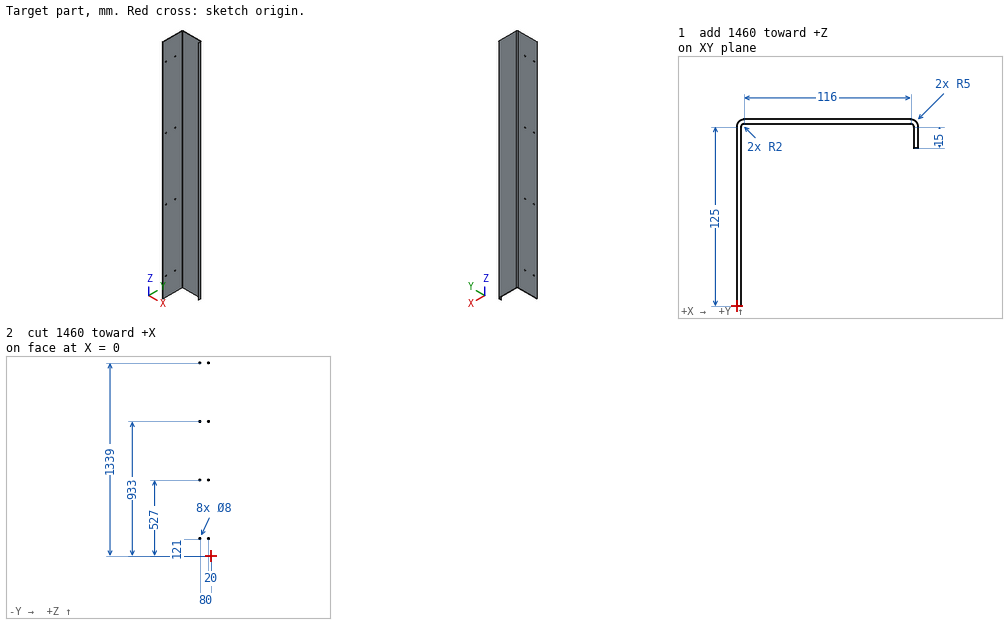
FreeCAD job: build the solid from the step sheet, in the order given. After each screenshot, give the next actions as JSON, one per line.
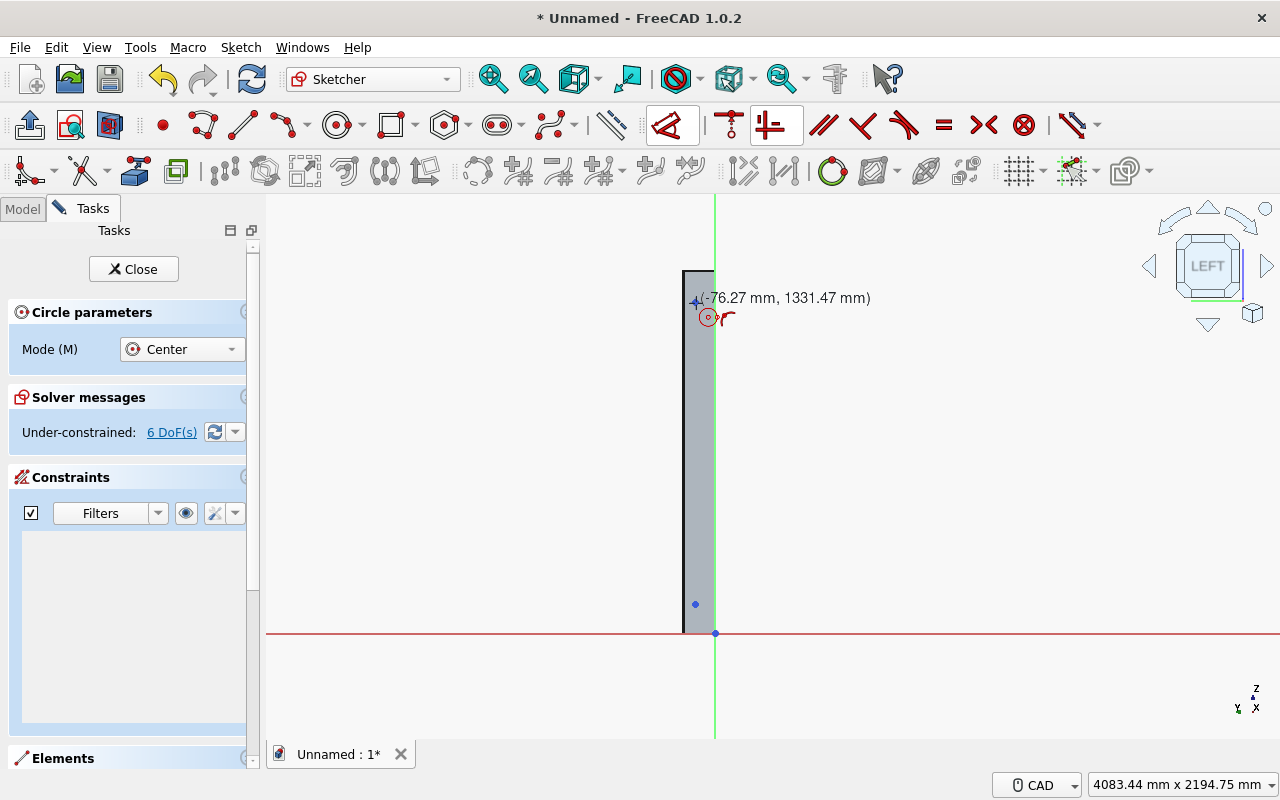
{"action": "scroll", "coordinate": [695, 402], "scroll_direction": "up", "scroll_amount": 16}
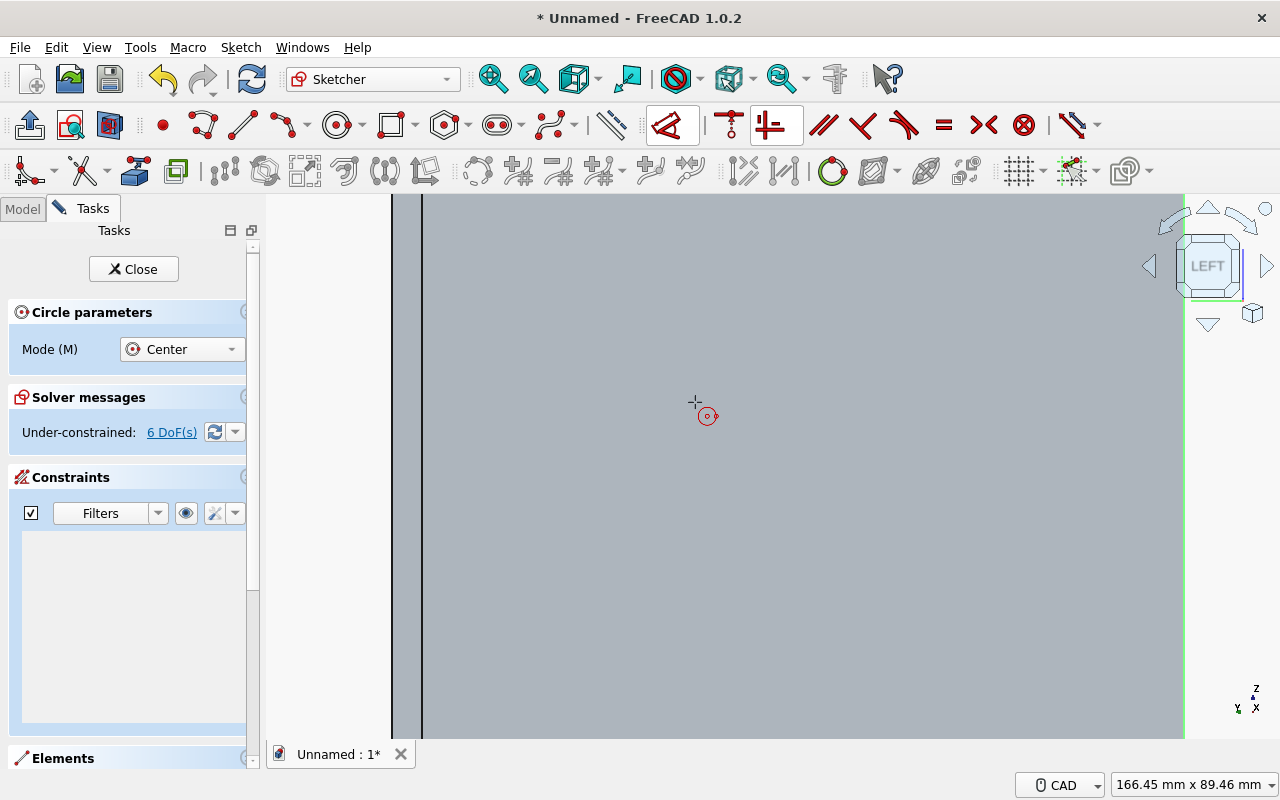
{"action": "scroll", "coordinate": [693, 387], "scroll_direction": "down", "scroll_amount": 15}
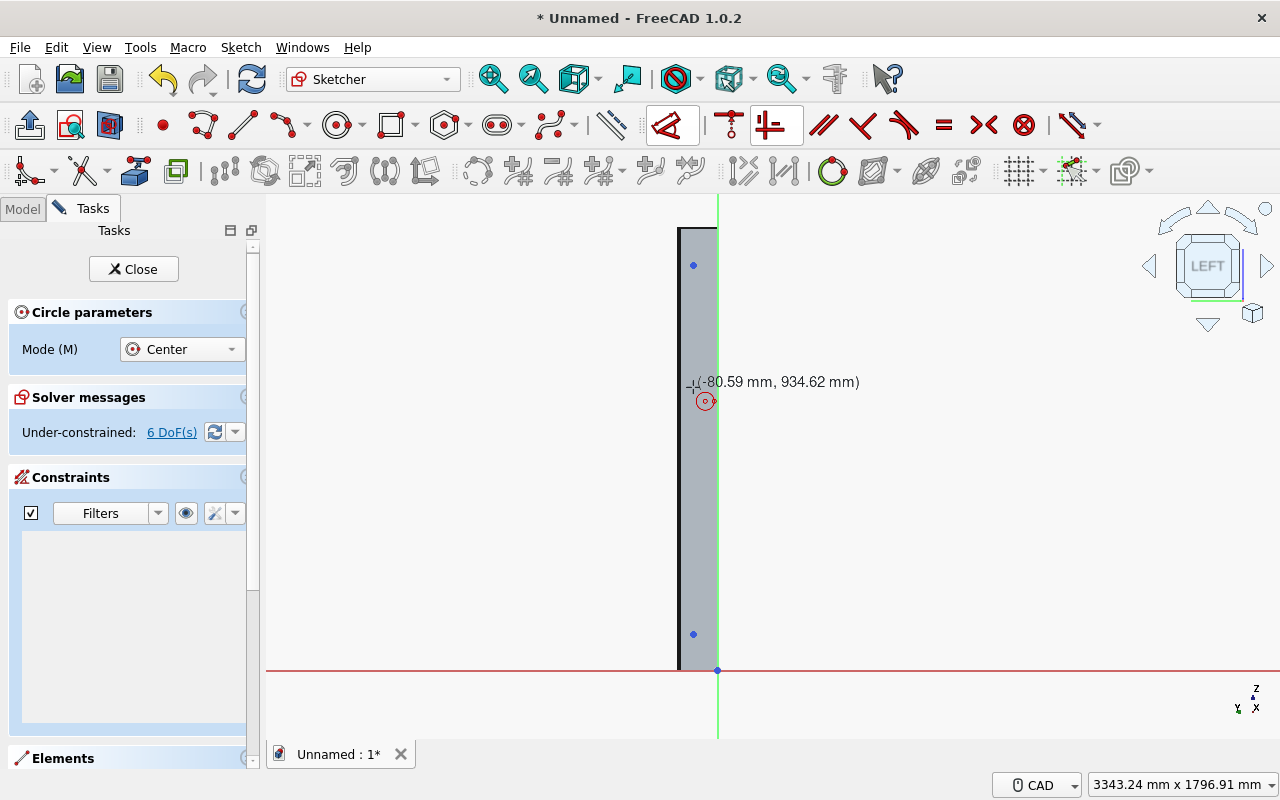
{"action": "left_click", "coordinate": [694, 388]}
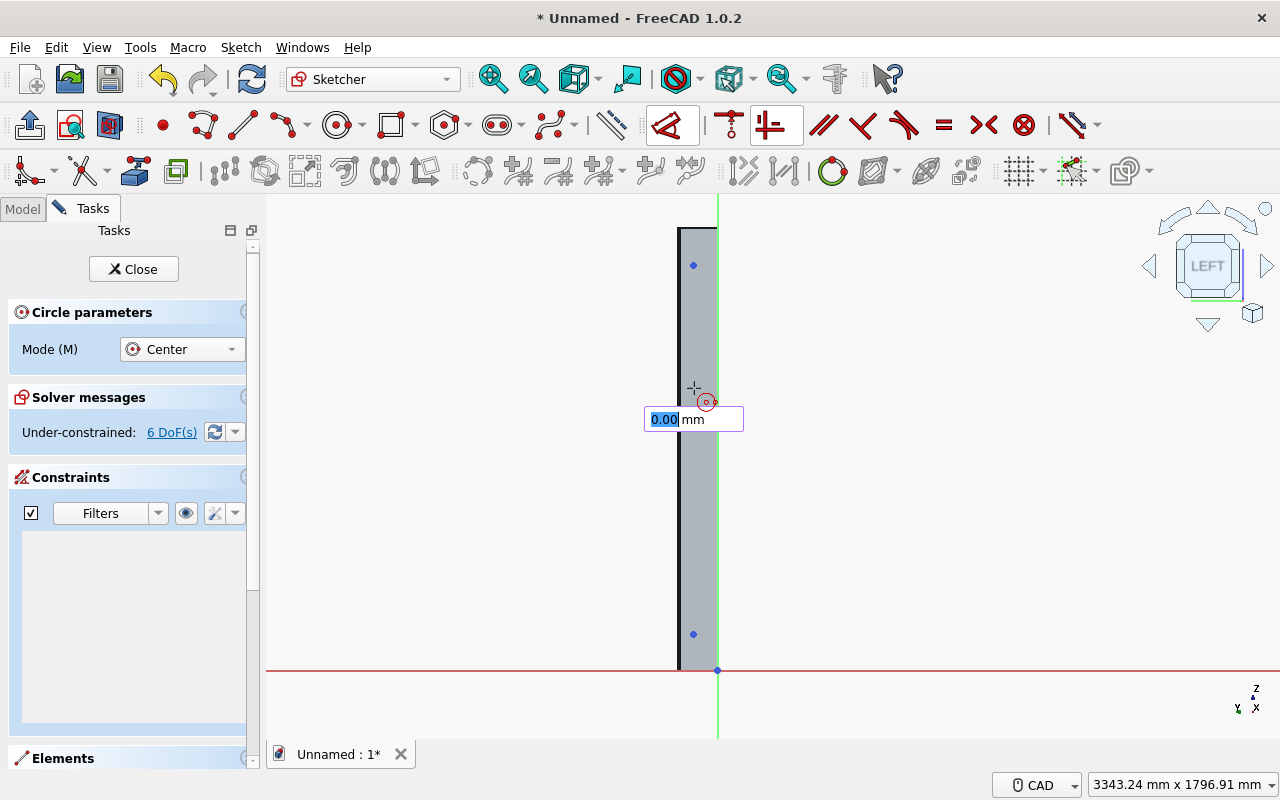
{"action": "scroll", "coordinate": [694, 387], "scroll_direction": "up", "scroll_amount": 13}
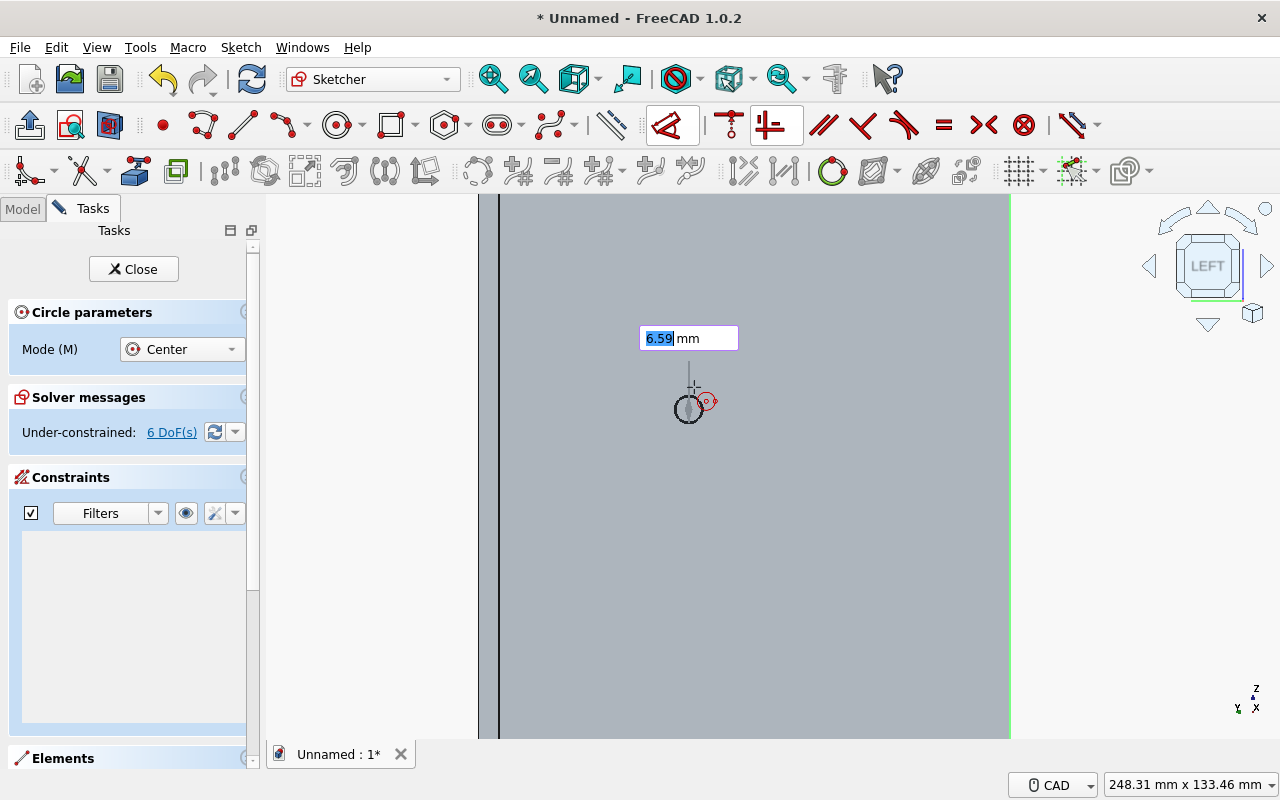
{"action": "left_click", "coordinate": [695, 383]}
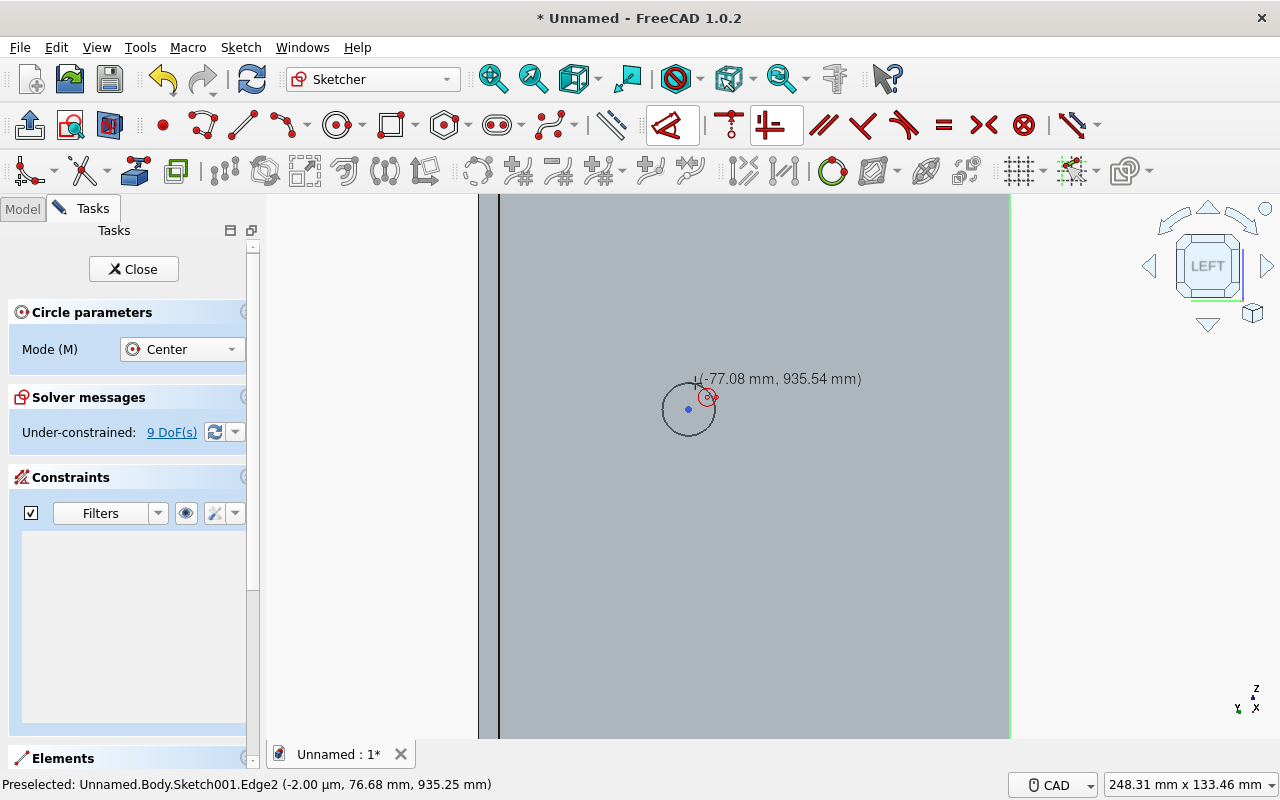
{"action": "scroll", "coordinate": [696, 402], "scroll_direction": "down", "scroll_amount": 14}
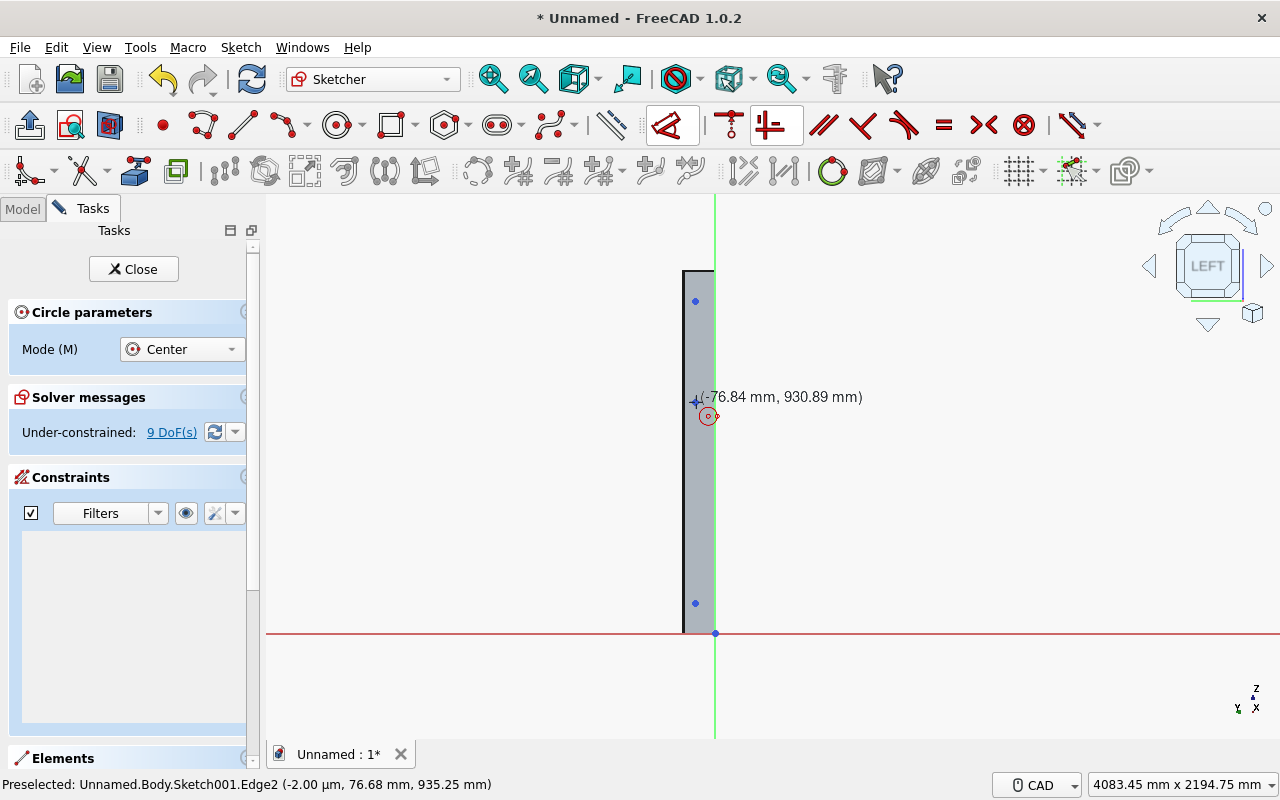
{"action": "scroll", "coordinate": [696, 503], "scroll_direction": "up", "scroll_amount": 16}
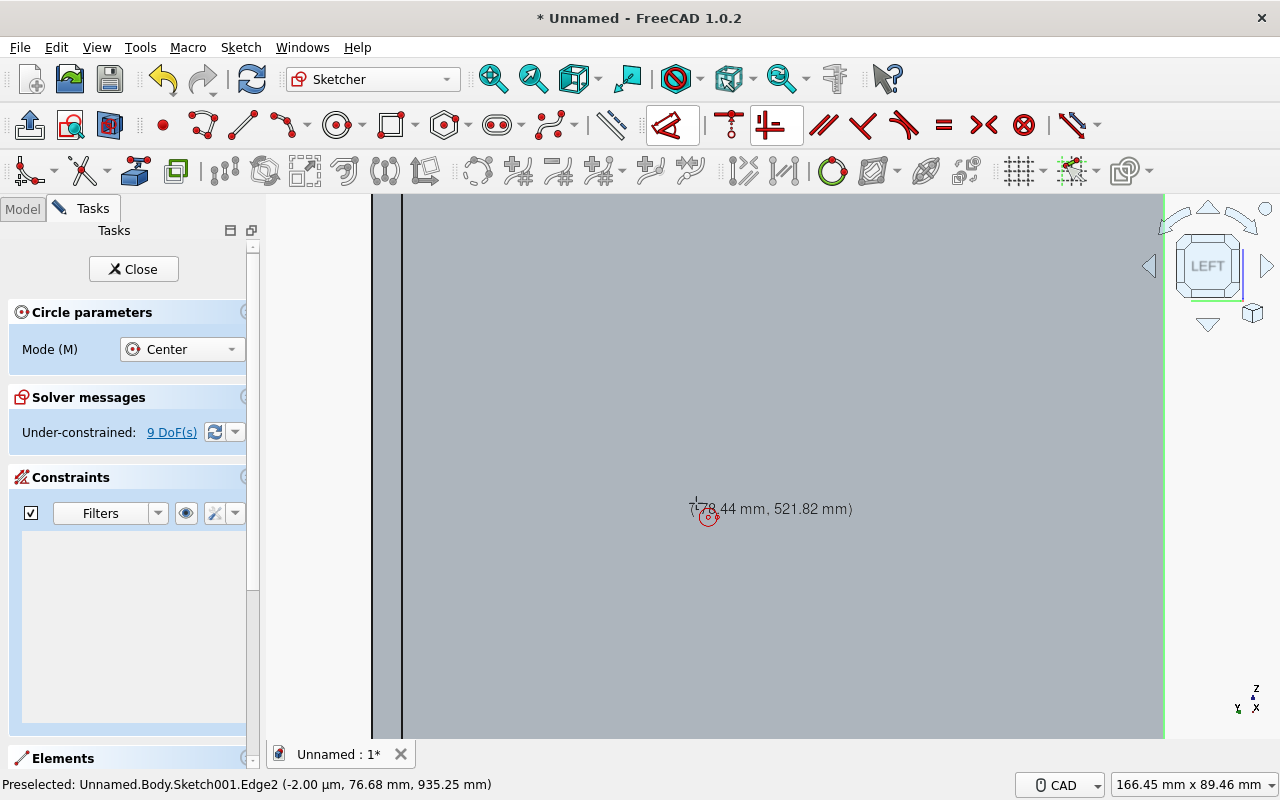
{"action": "scroll", "coordinate": [694, 512], "scroll_direction": "down", "scroll_amount": 15}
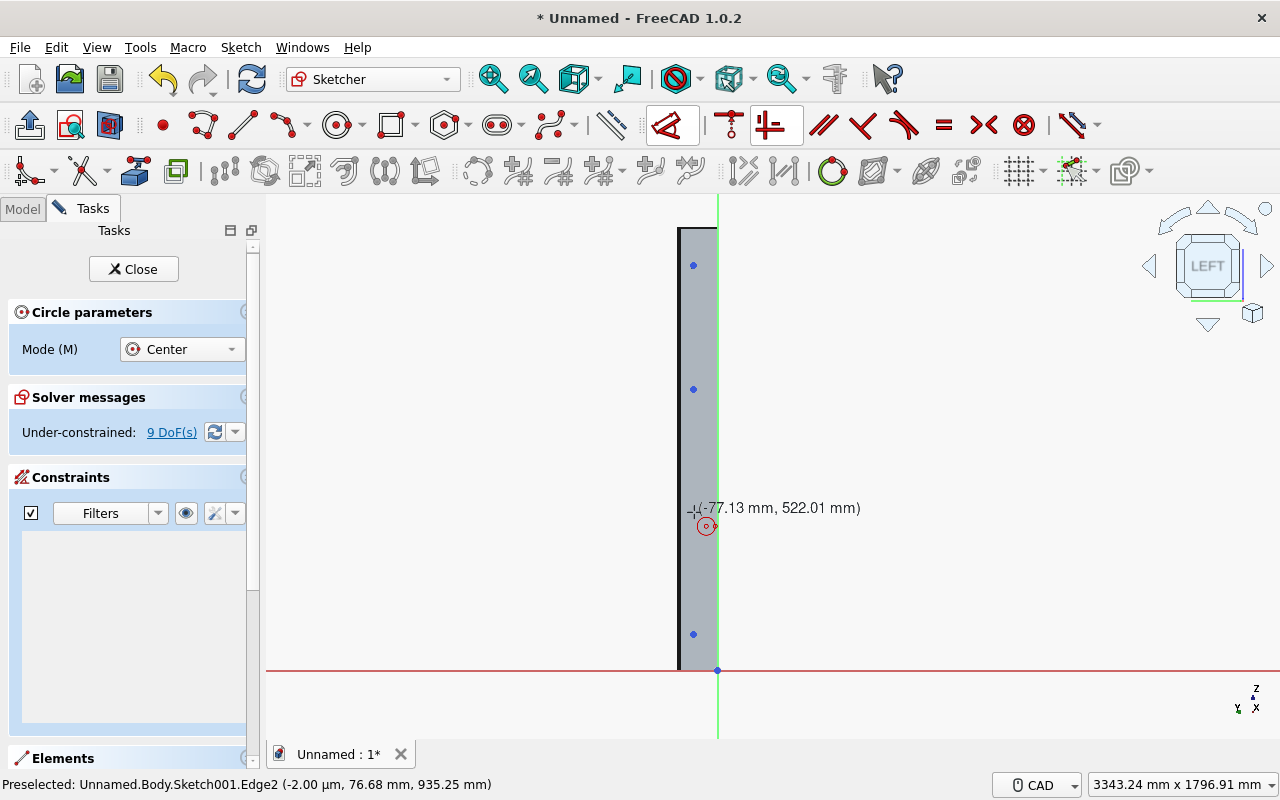
{"action": "left_click", "coordinate": [694, 511]}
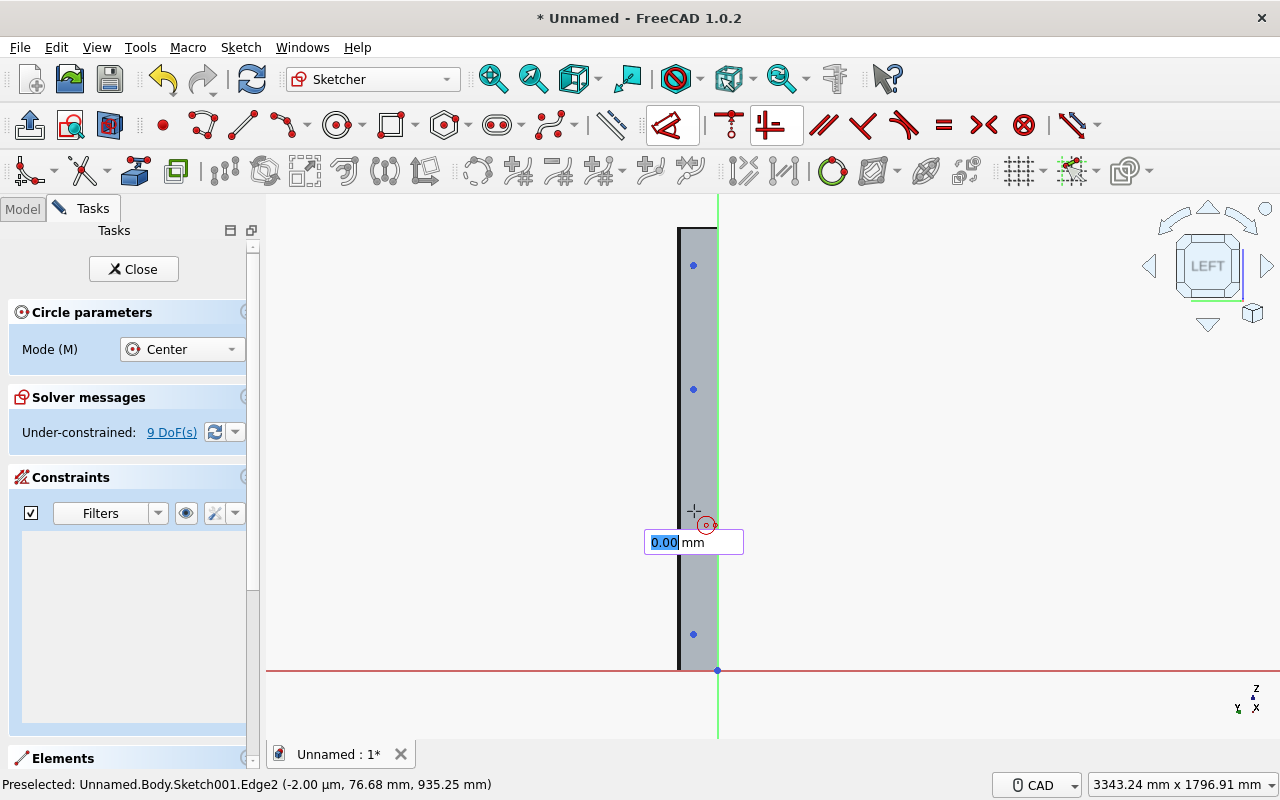
{"action": "scroll", "coordinate": [694, 510], "scroll_direction": "up", "scroll_amount": 13}